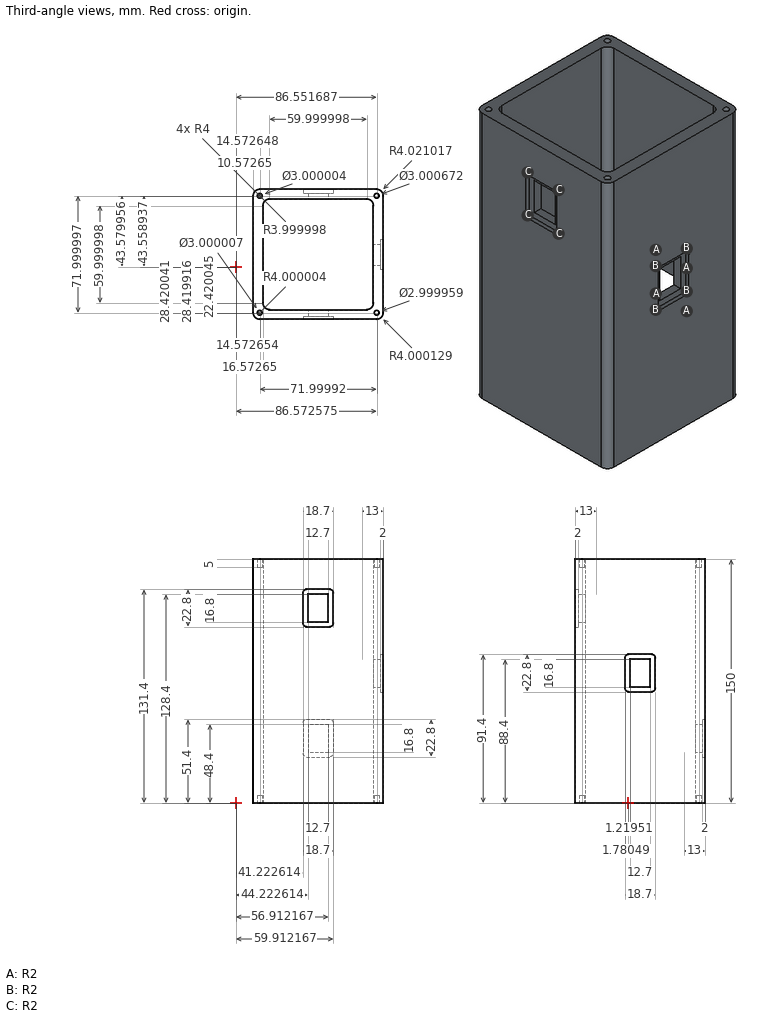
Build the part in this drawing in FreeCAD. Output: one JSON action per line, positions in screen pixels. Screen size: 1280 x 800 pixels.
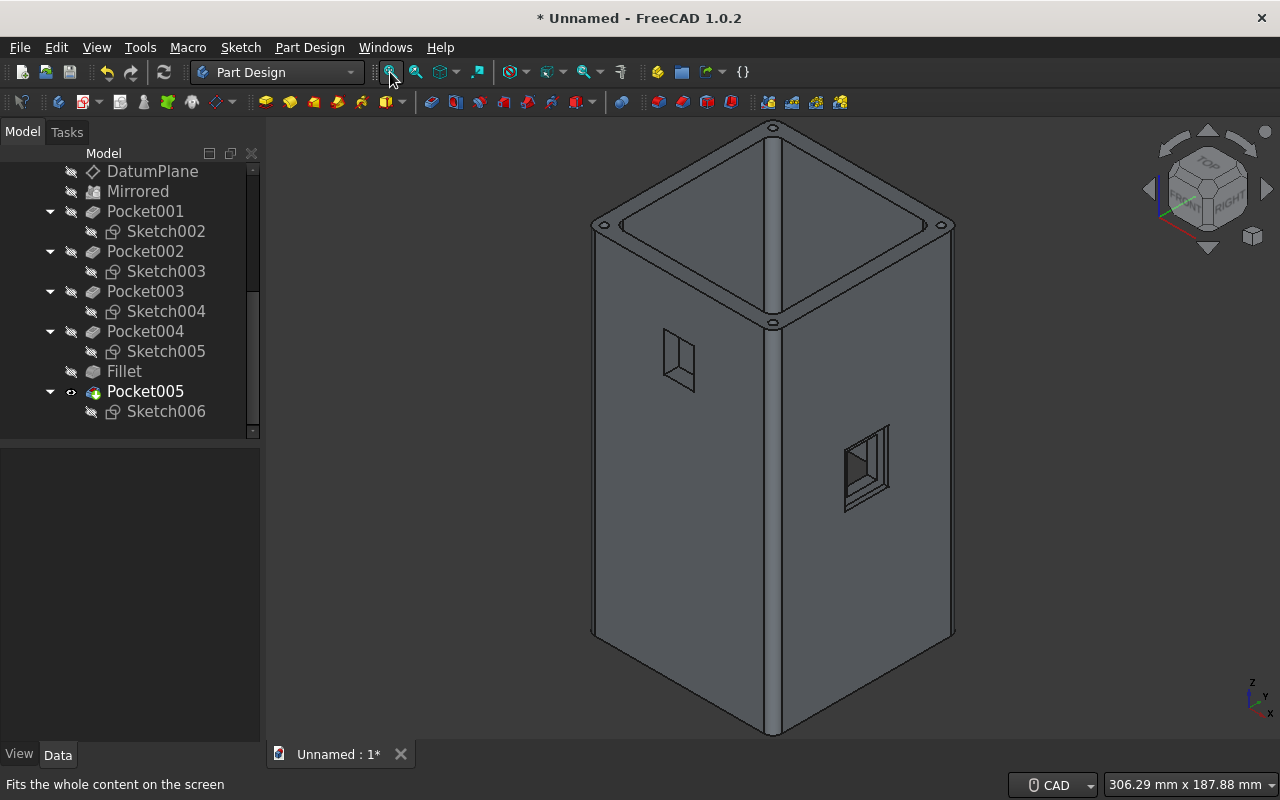
{"action": "scroll", "coordinate": [886, 423], "scroll_direction": "up", "scroll_amount": 9}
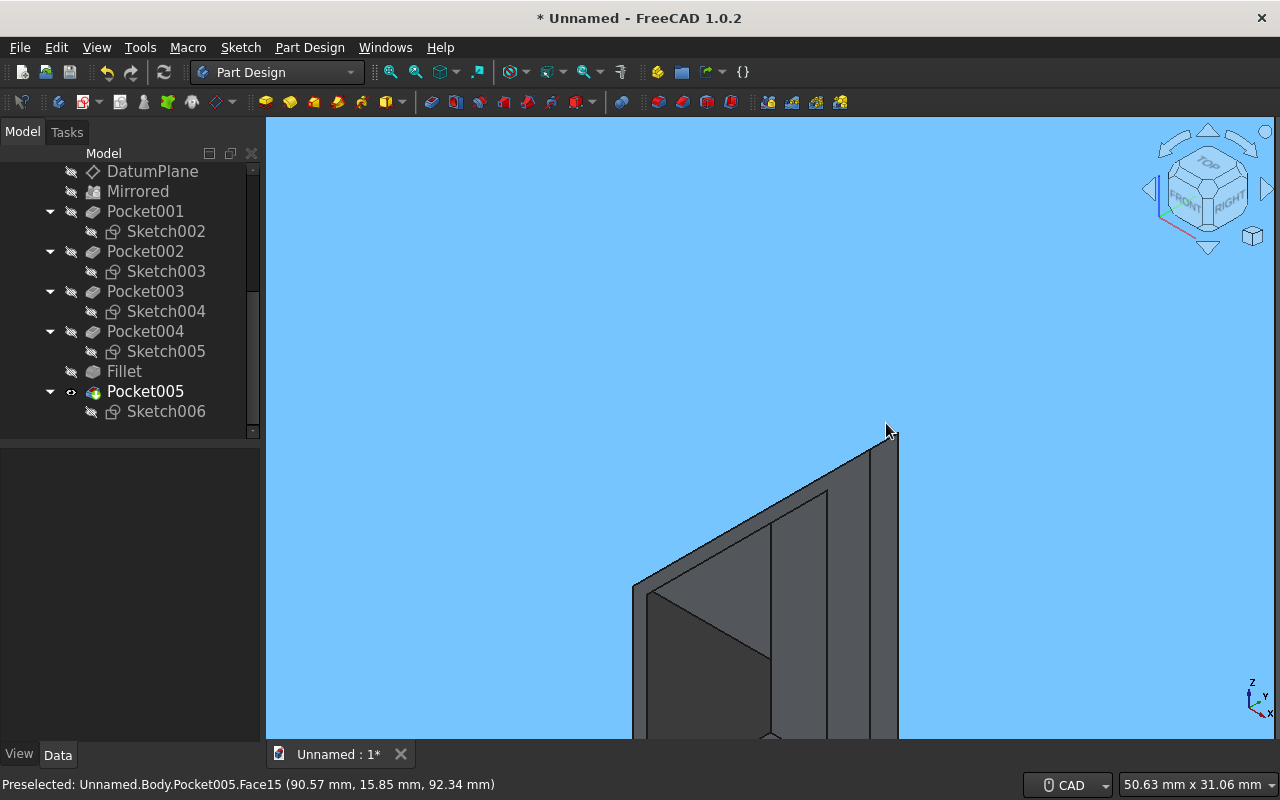
{"action": "key", "text": "v f"}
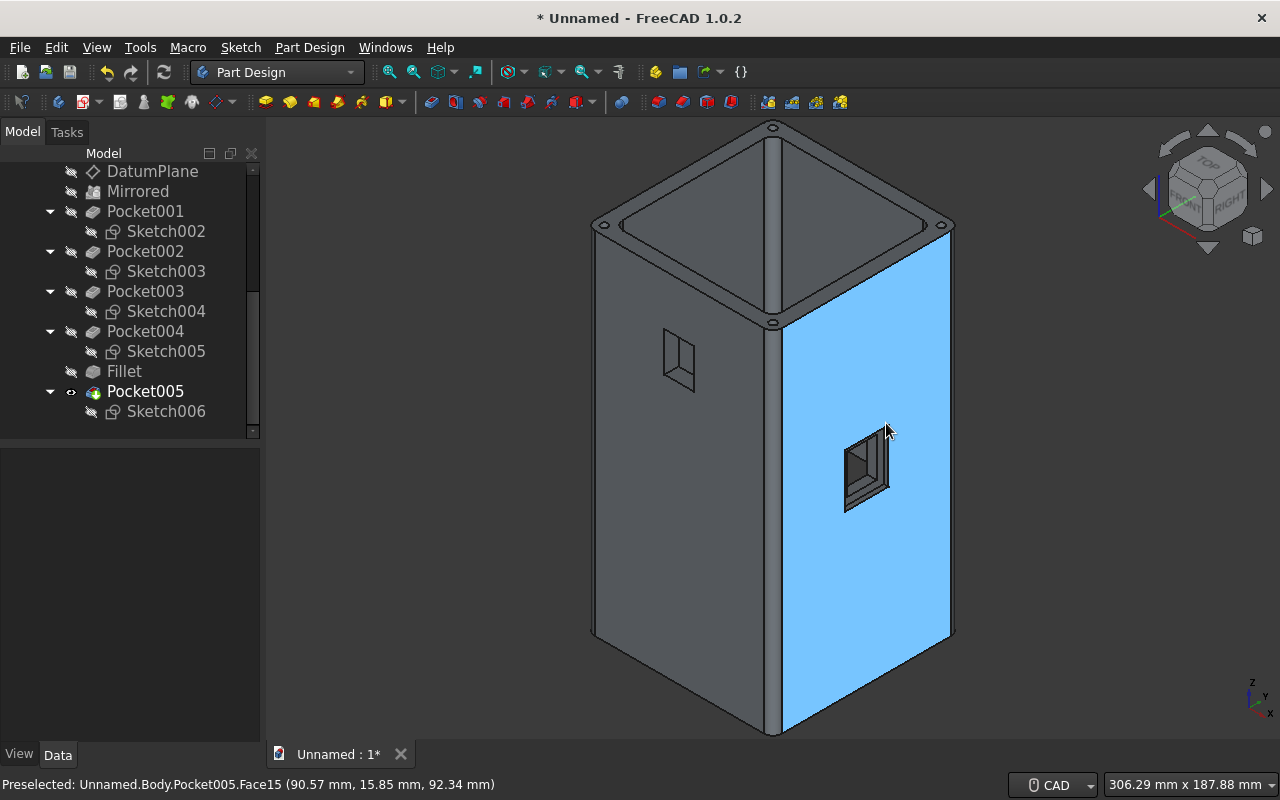
{"action": "key", "text": "1"}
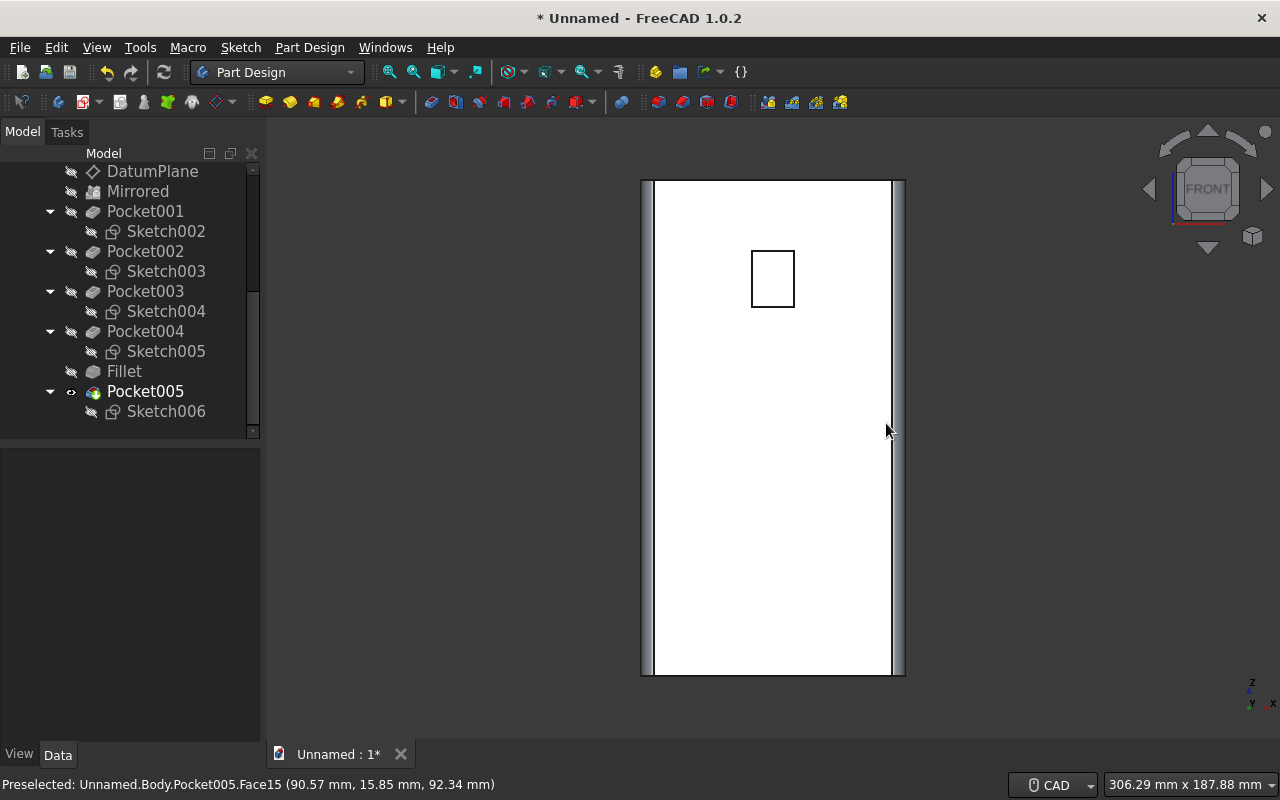
{"action": "scroll", "coordinate": [902, 373], "scroll_direction": "up", "scroll_amount": 9}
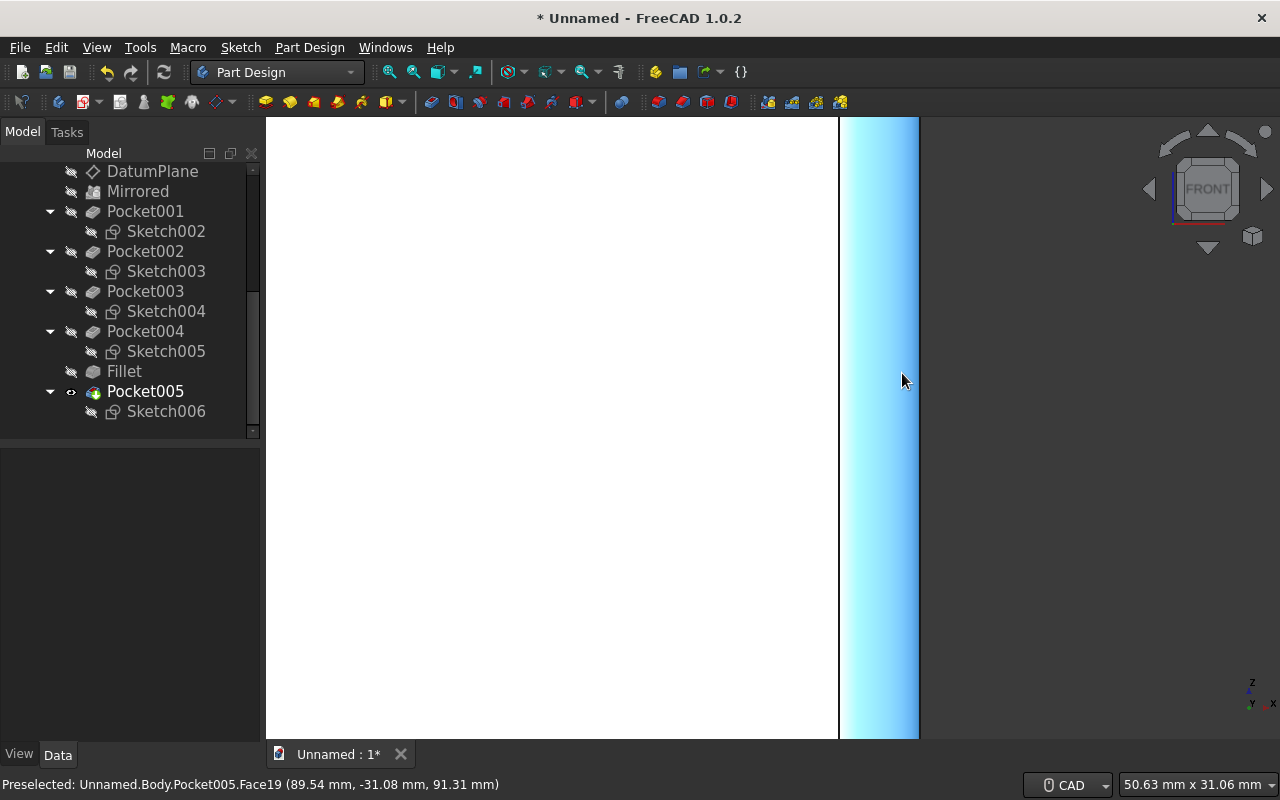
{"action": "key", "text": "v f"}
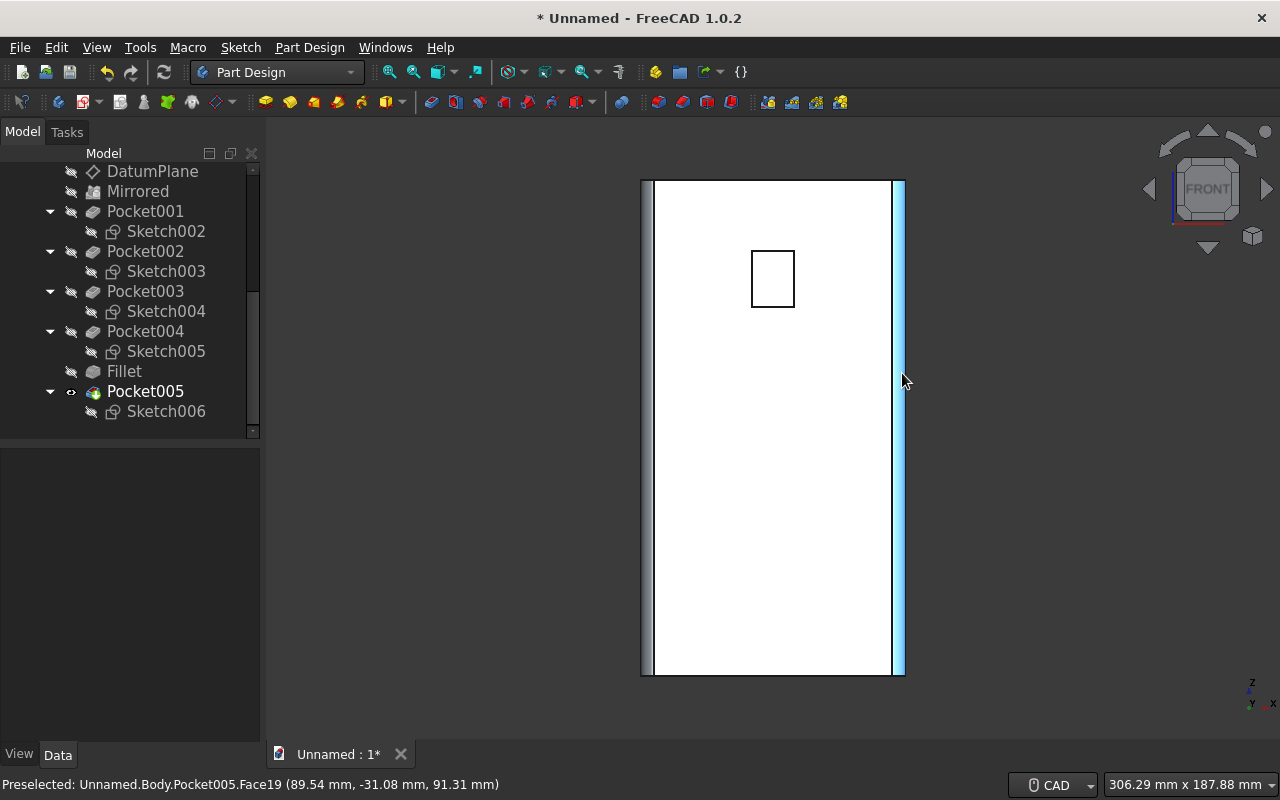
{"action": "key", "text": "3"}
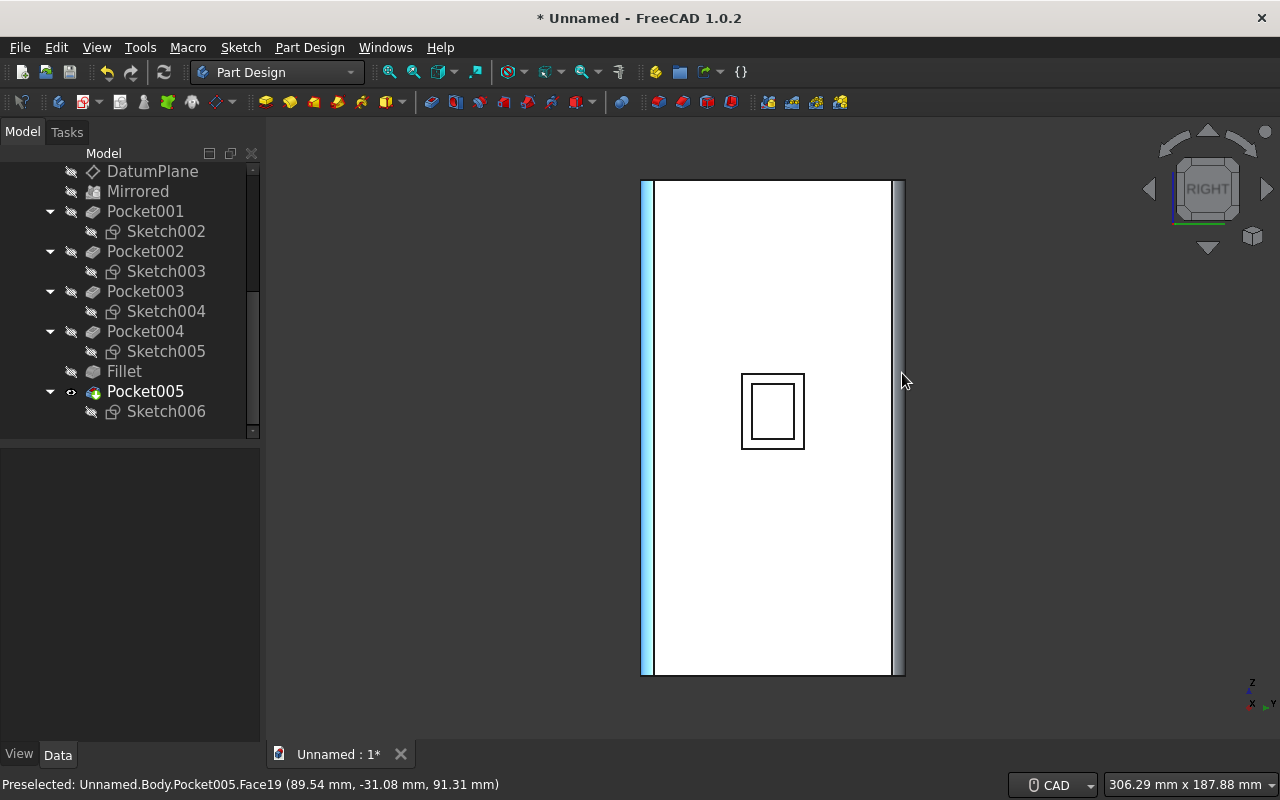
{"action": "scroll", "coordinate": [804, 373], "scroll_direction": "up", "scroll_amount": 9}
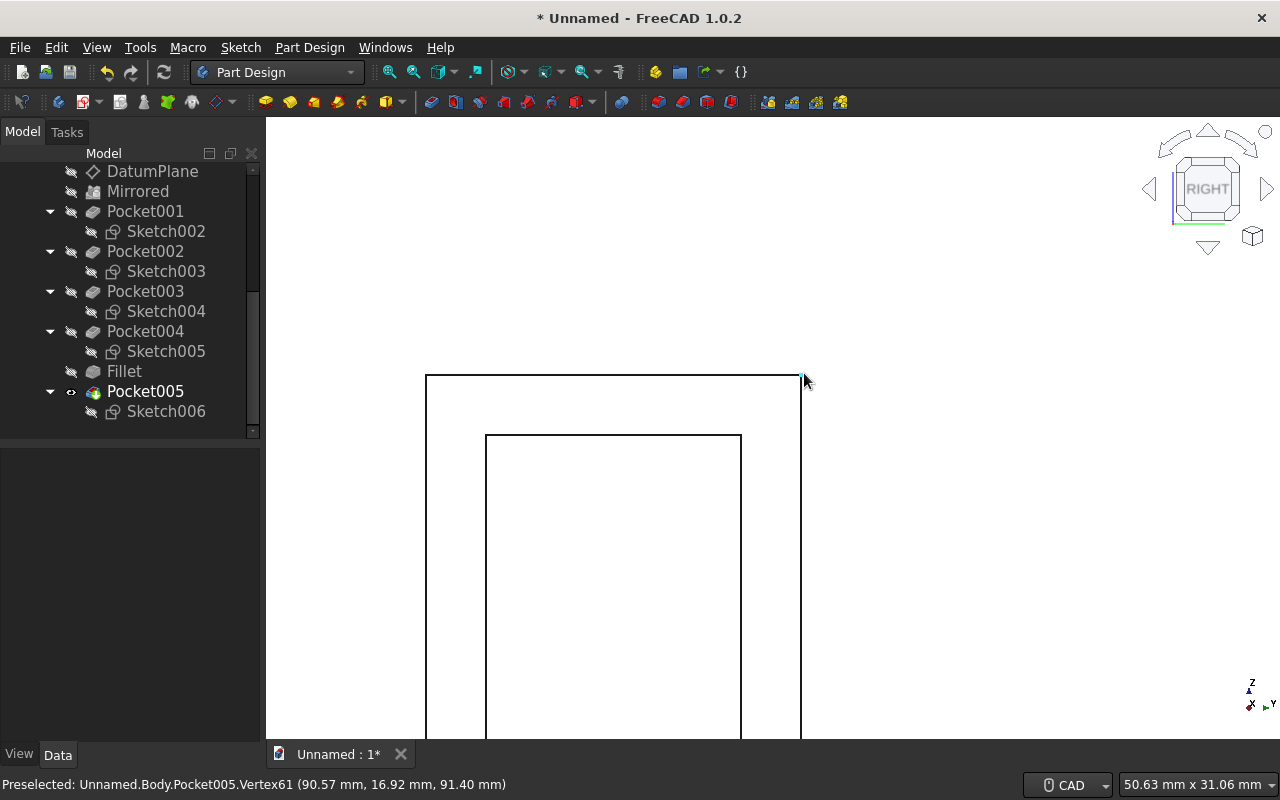
{"action": "left_click", "coordinate": [390, 72]}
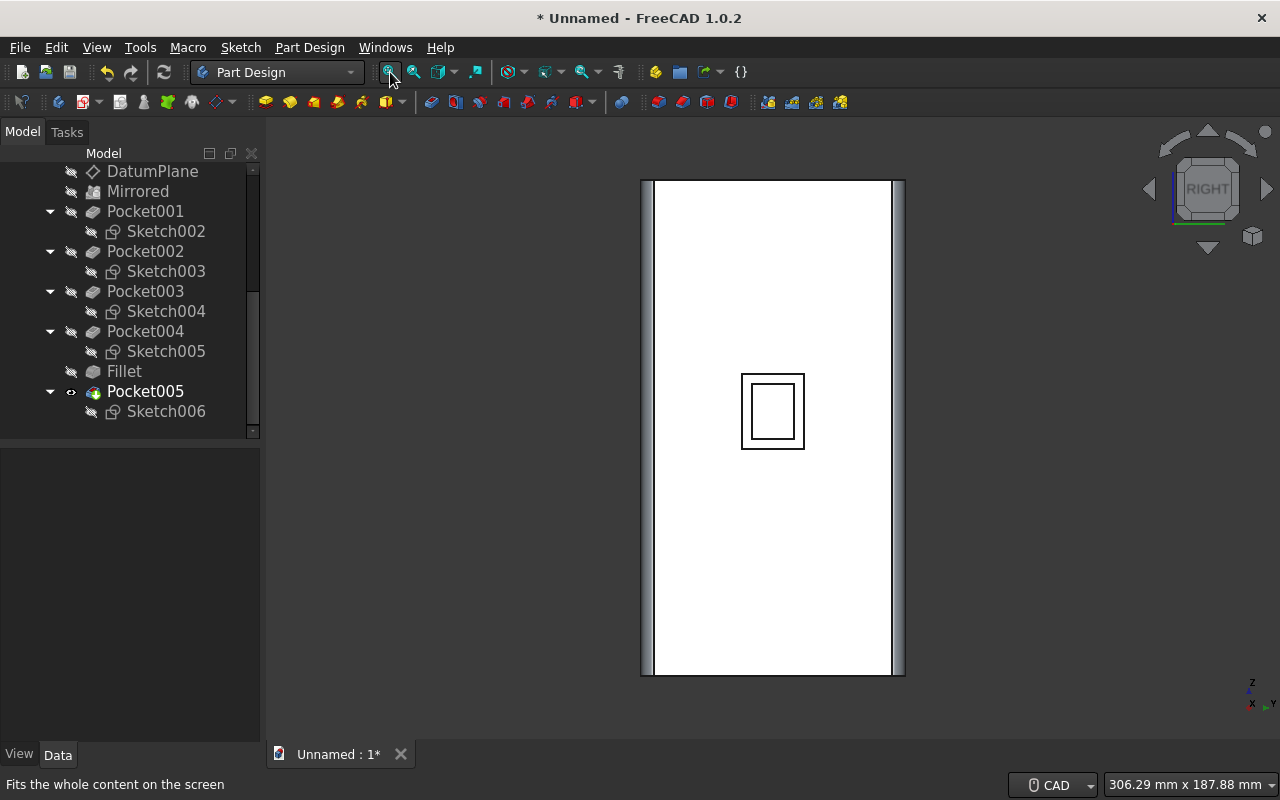
{"action": "key", "text": "5"}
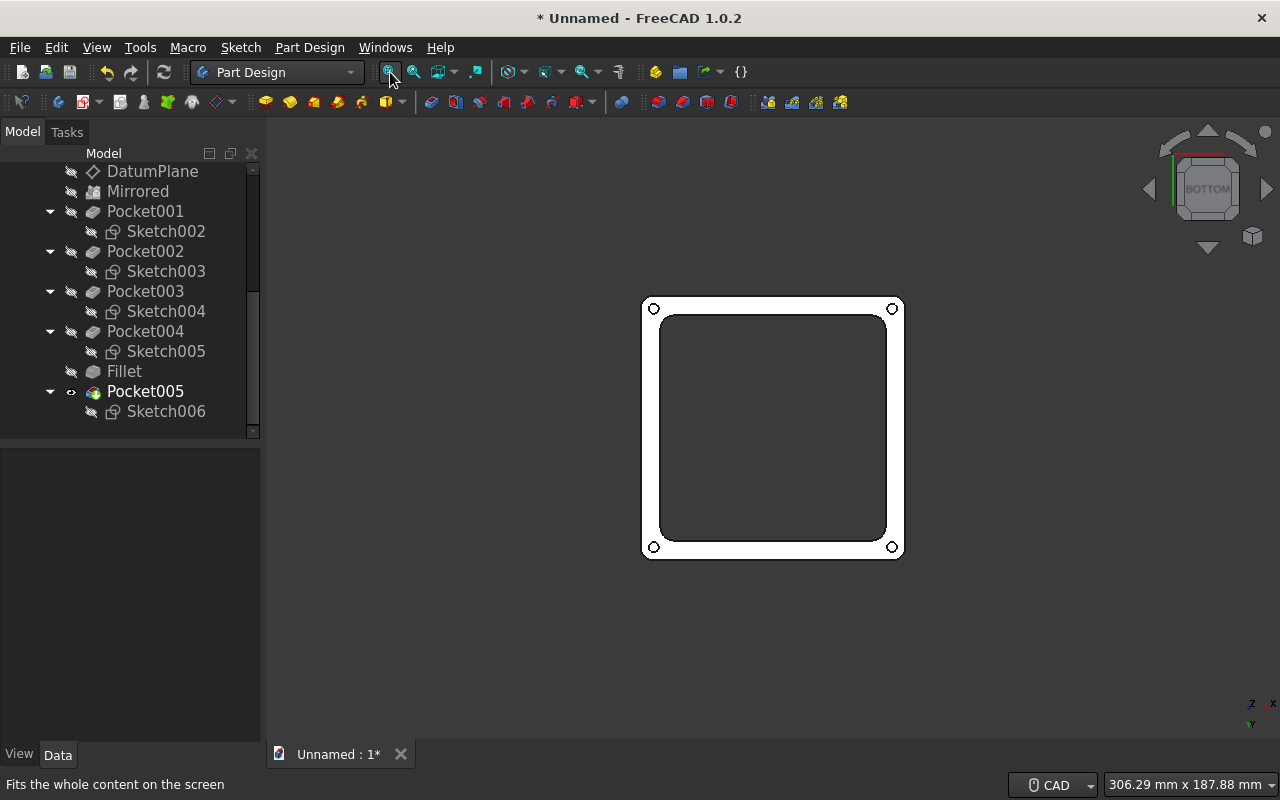
{"action": "left_click", "coordinate": [390, 72]}